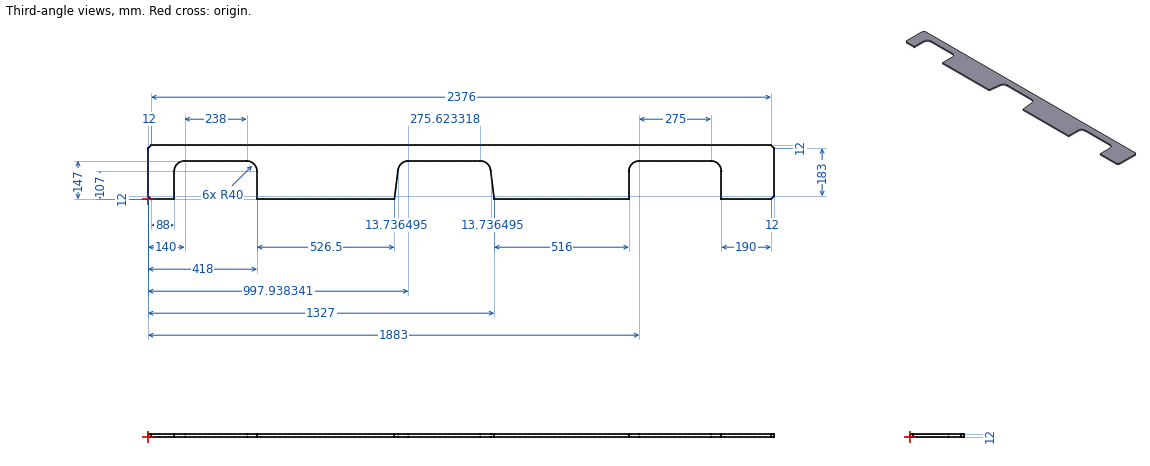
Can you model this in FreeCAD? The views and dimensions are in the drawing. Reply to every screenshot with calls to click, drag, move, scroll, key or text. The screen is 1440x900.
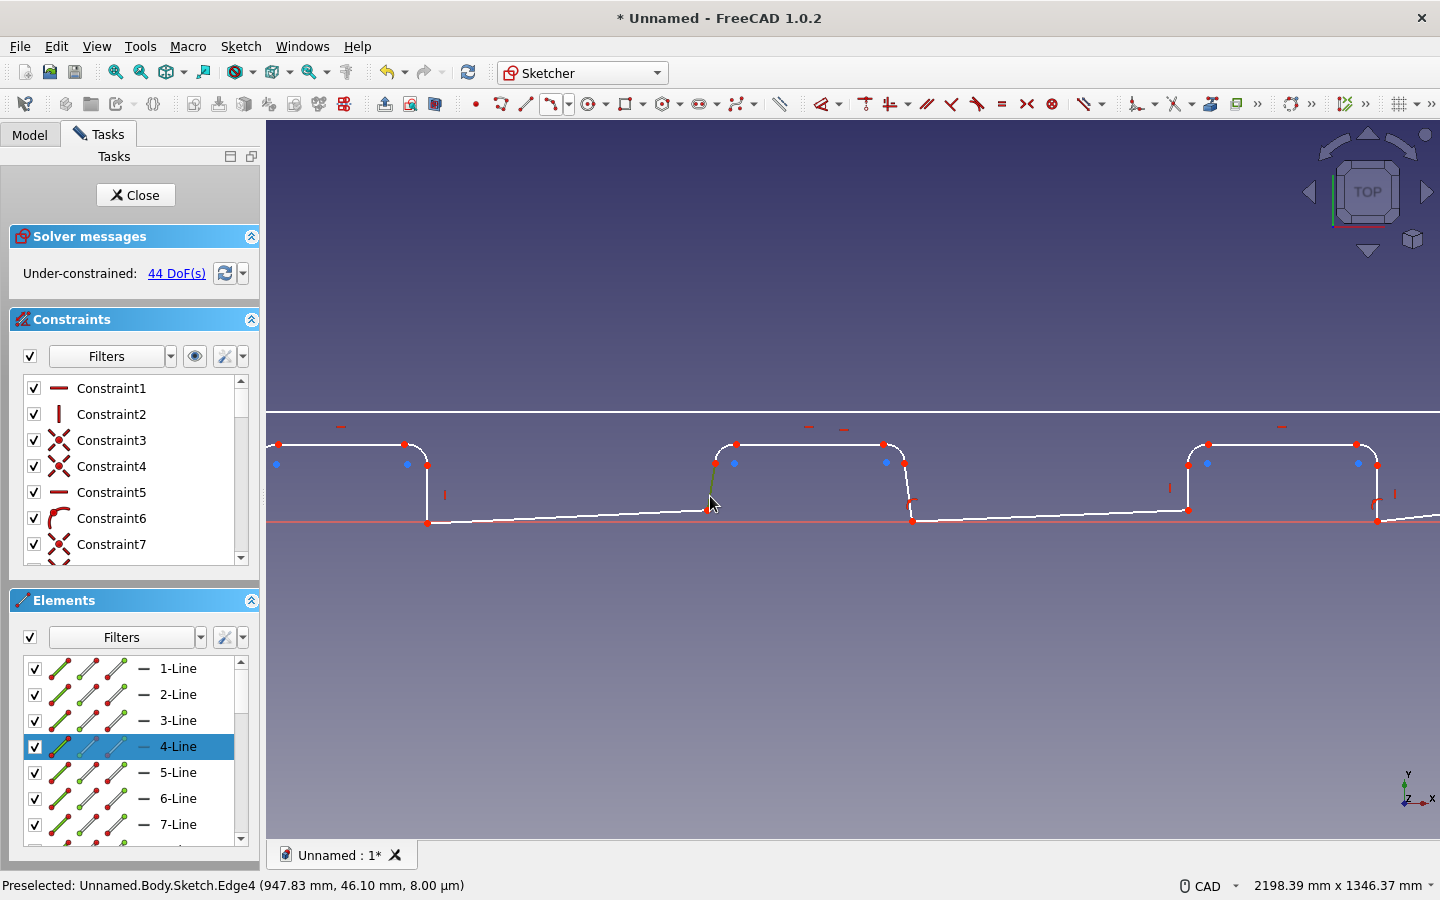
scroll(727, 446, up, 2)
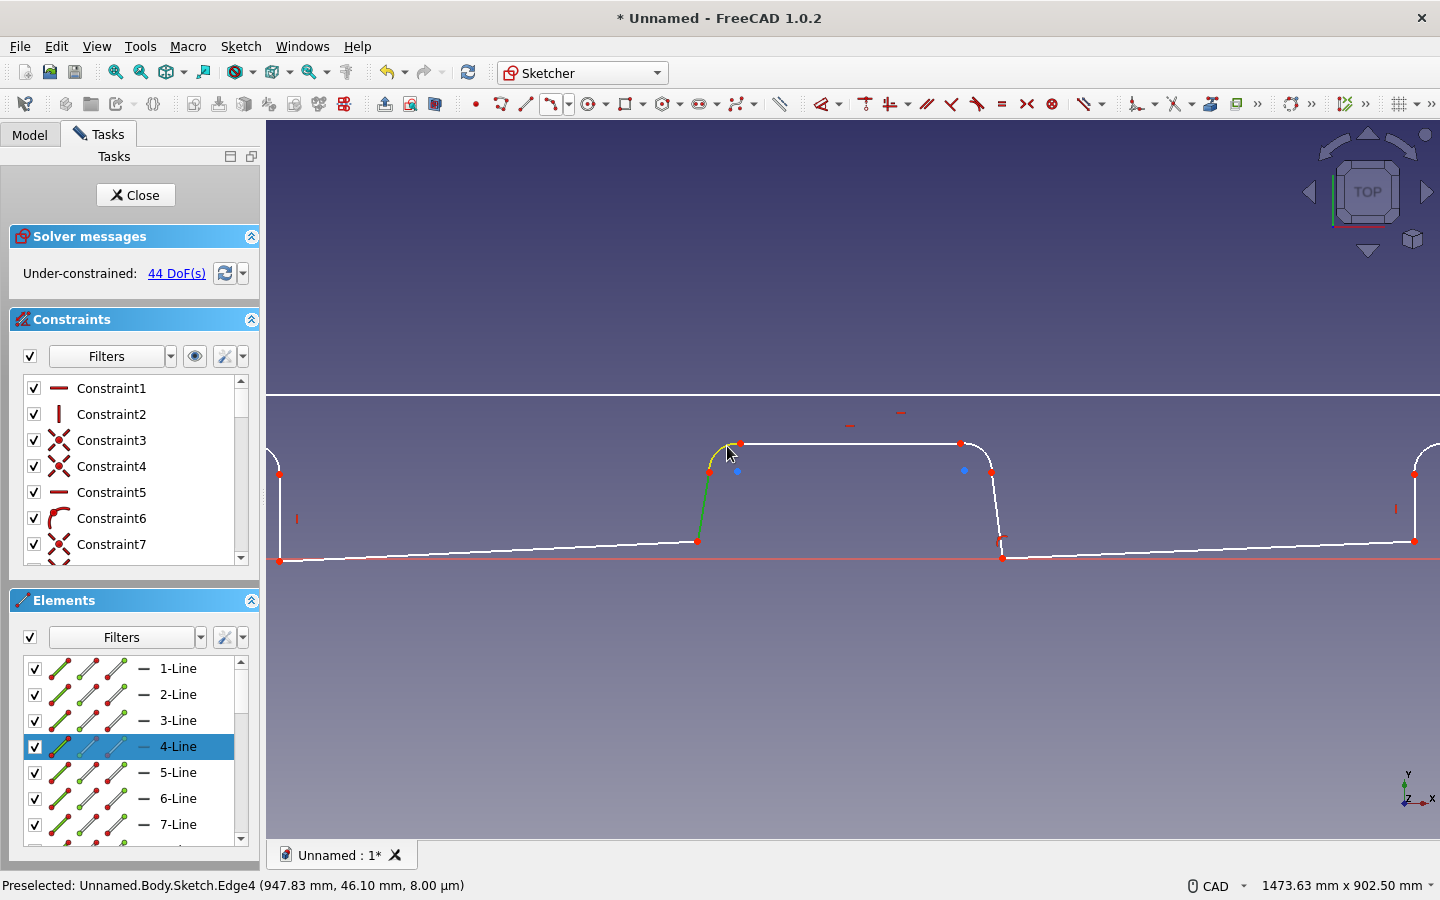
click(726, 446)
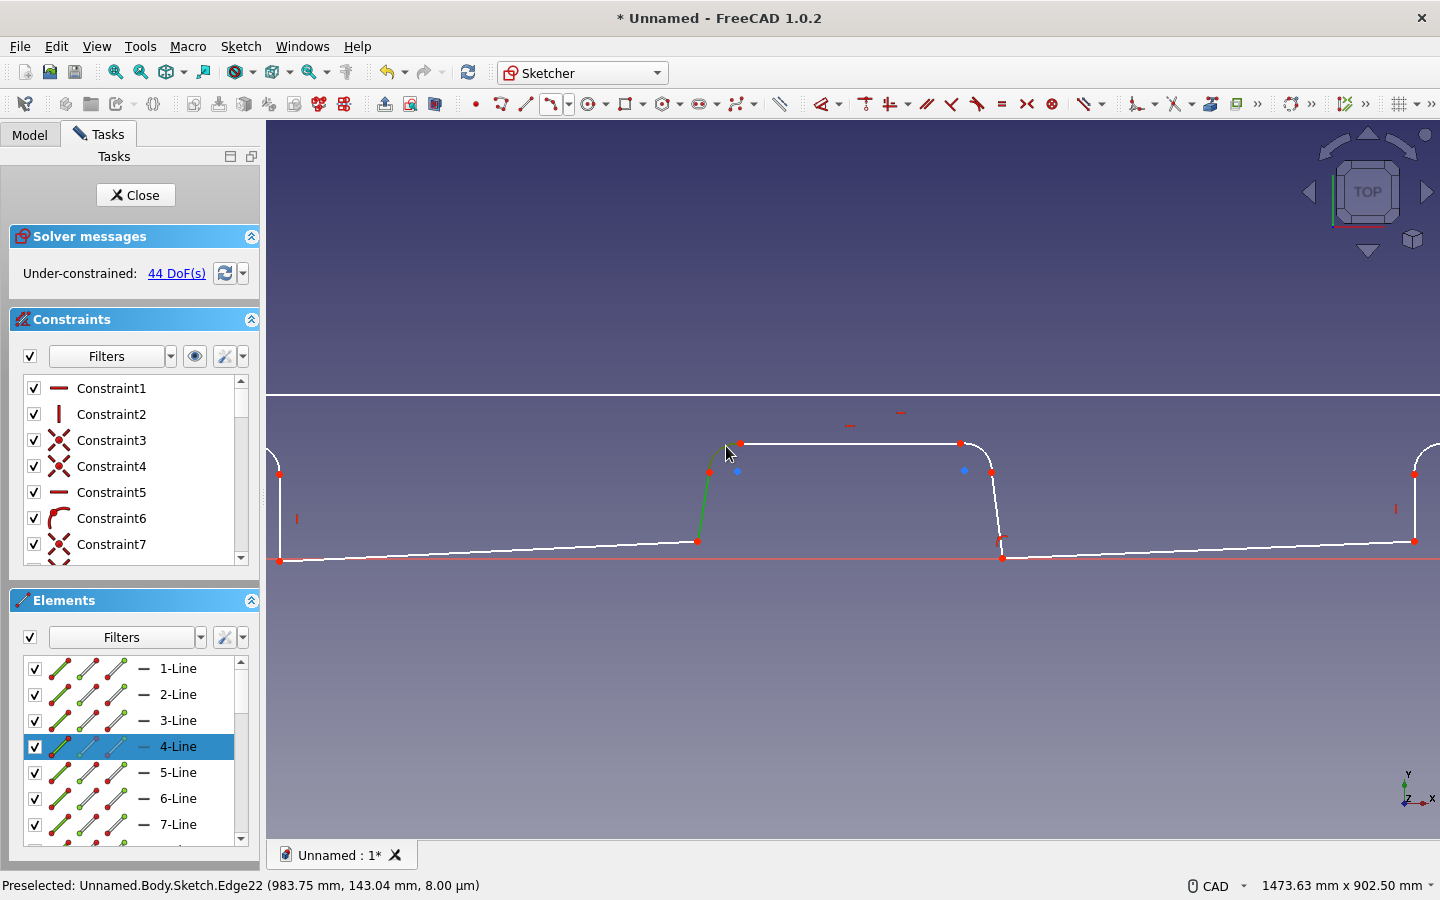
click(977, 104)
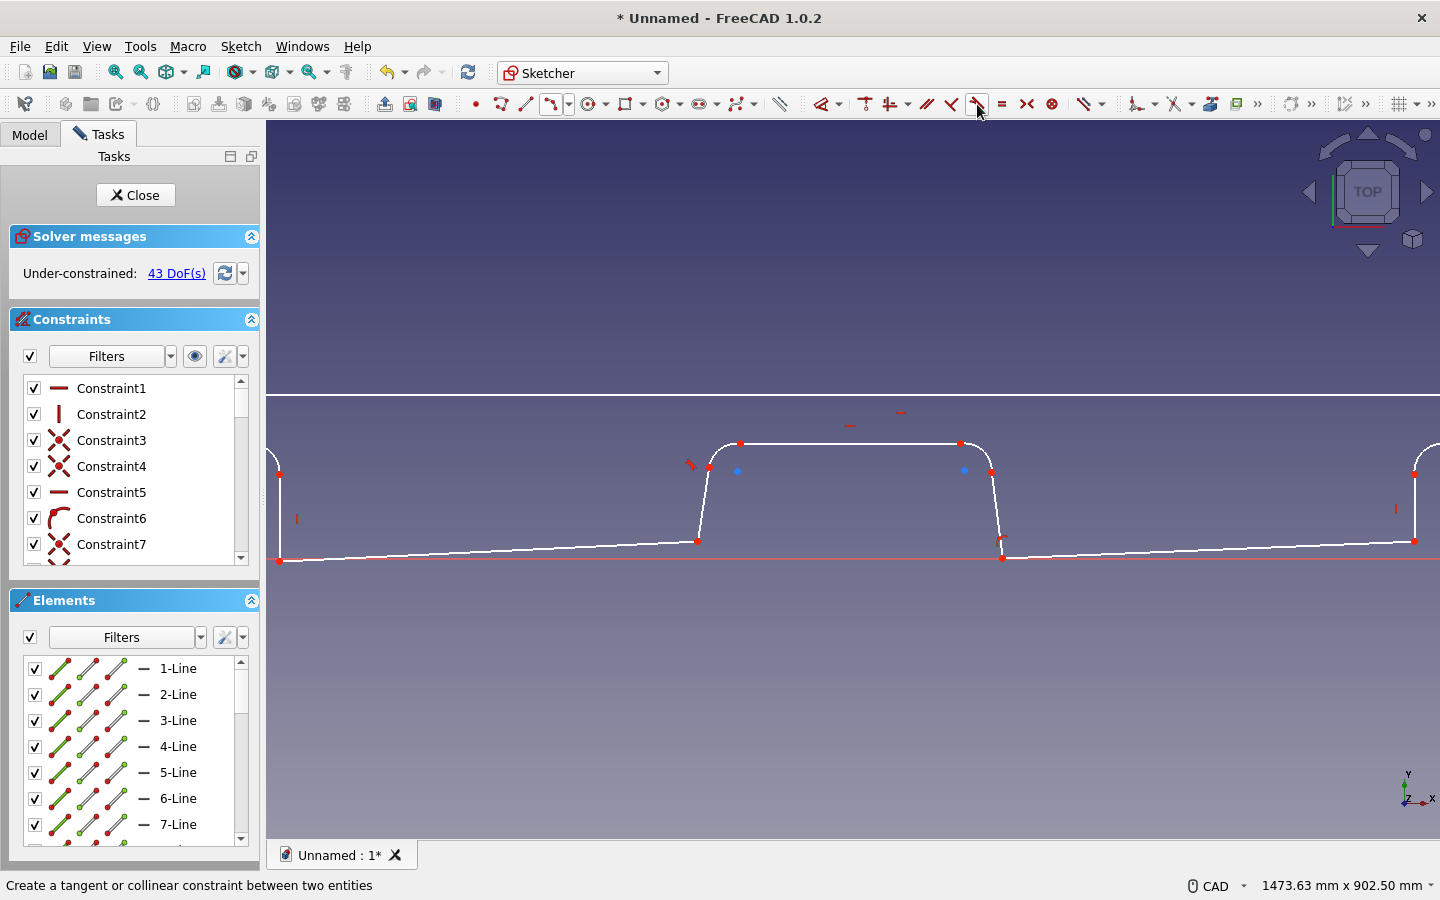
click(995, 498)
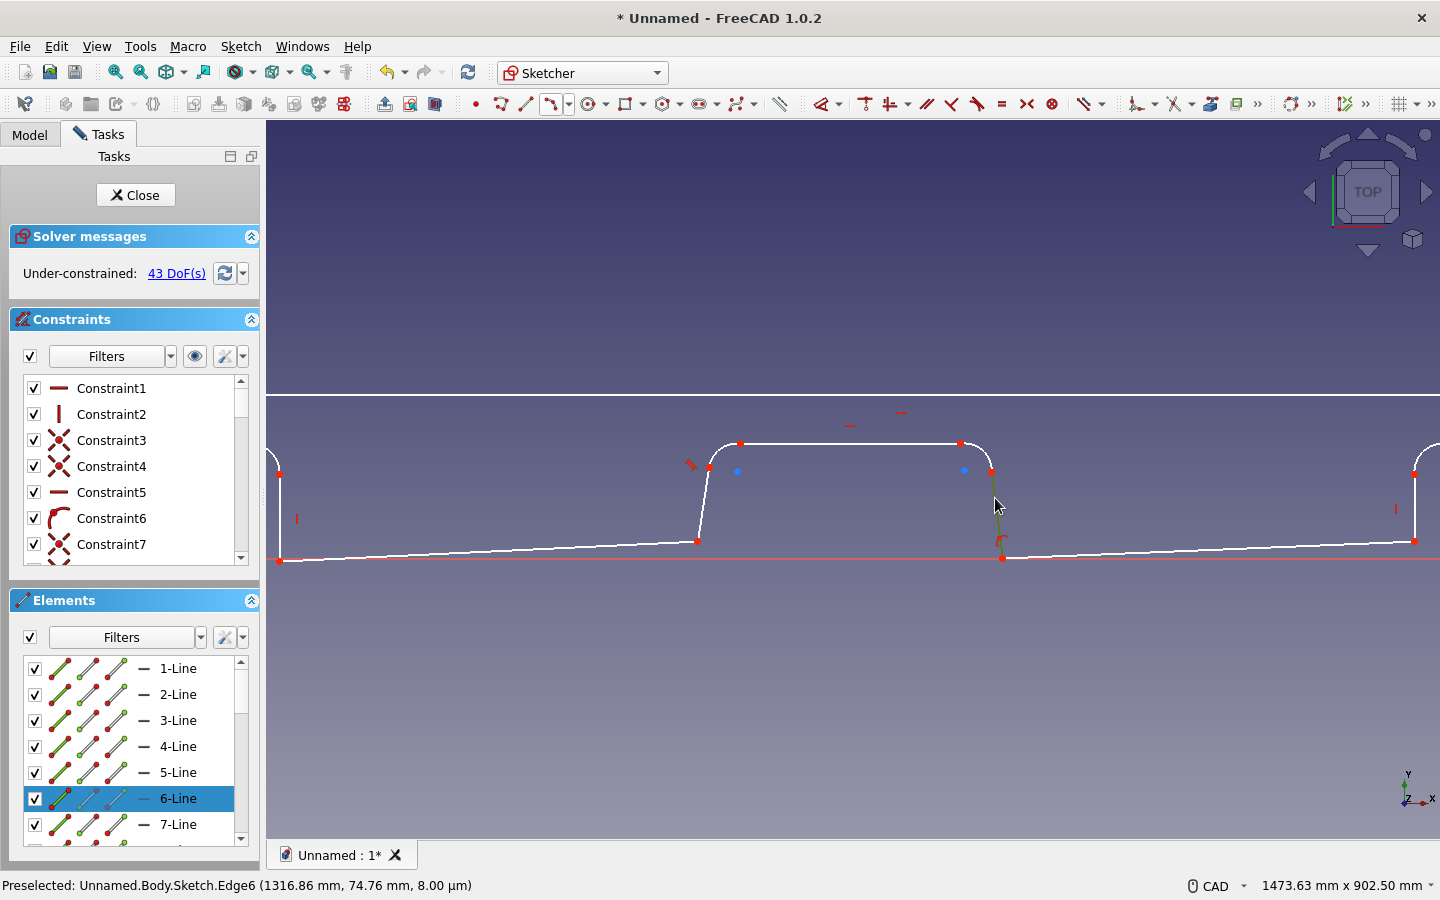
click(989, 458)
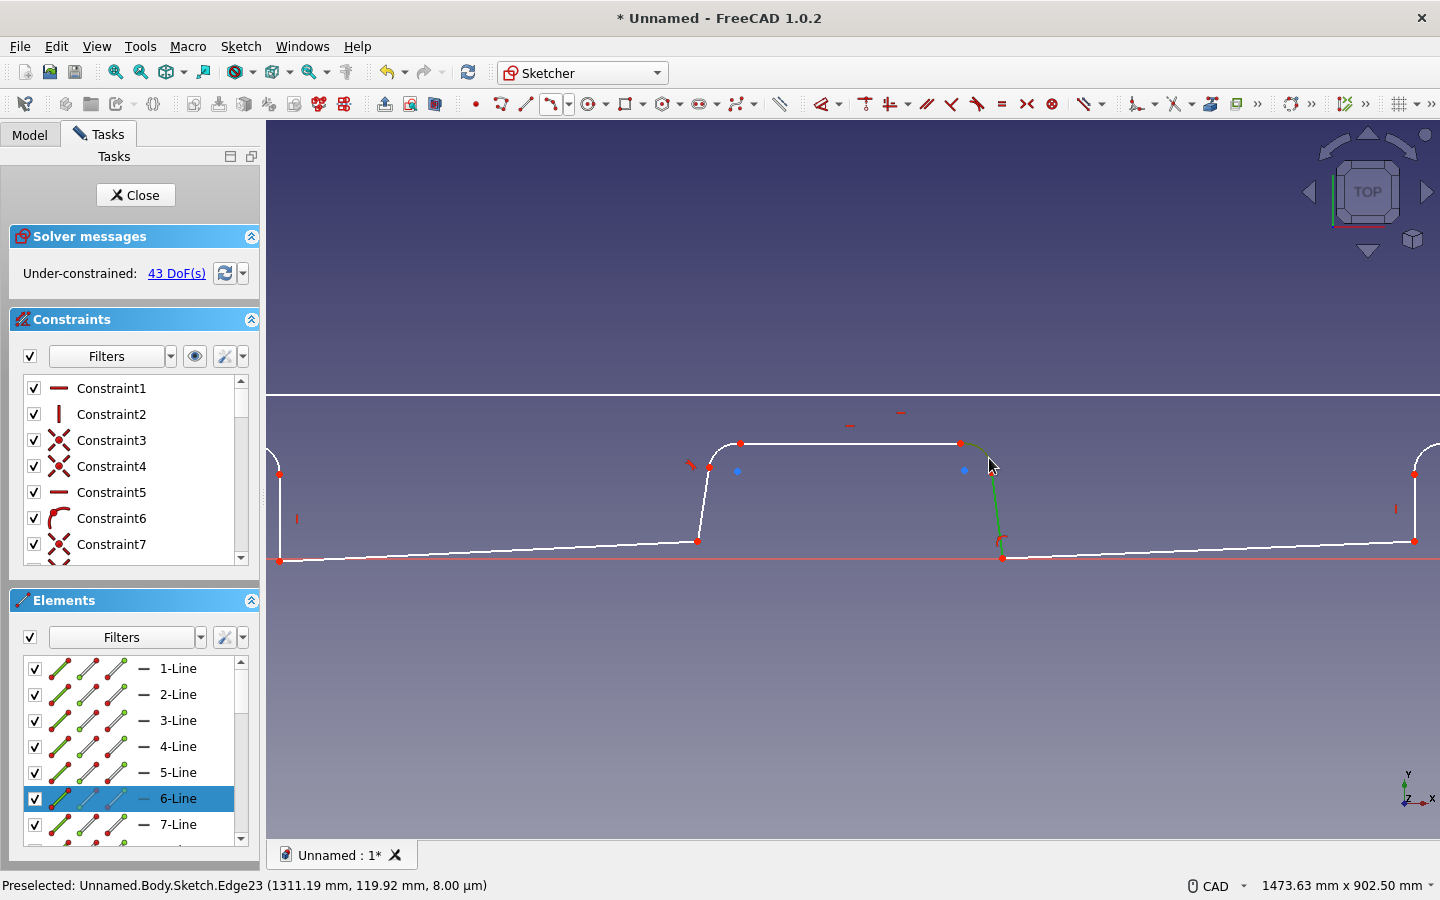
click(977, 104)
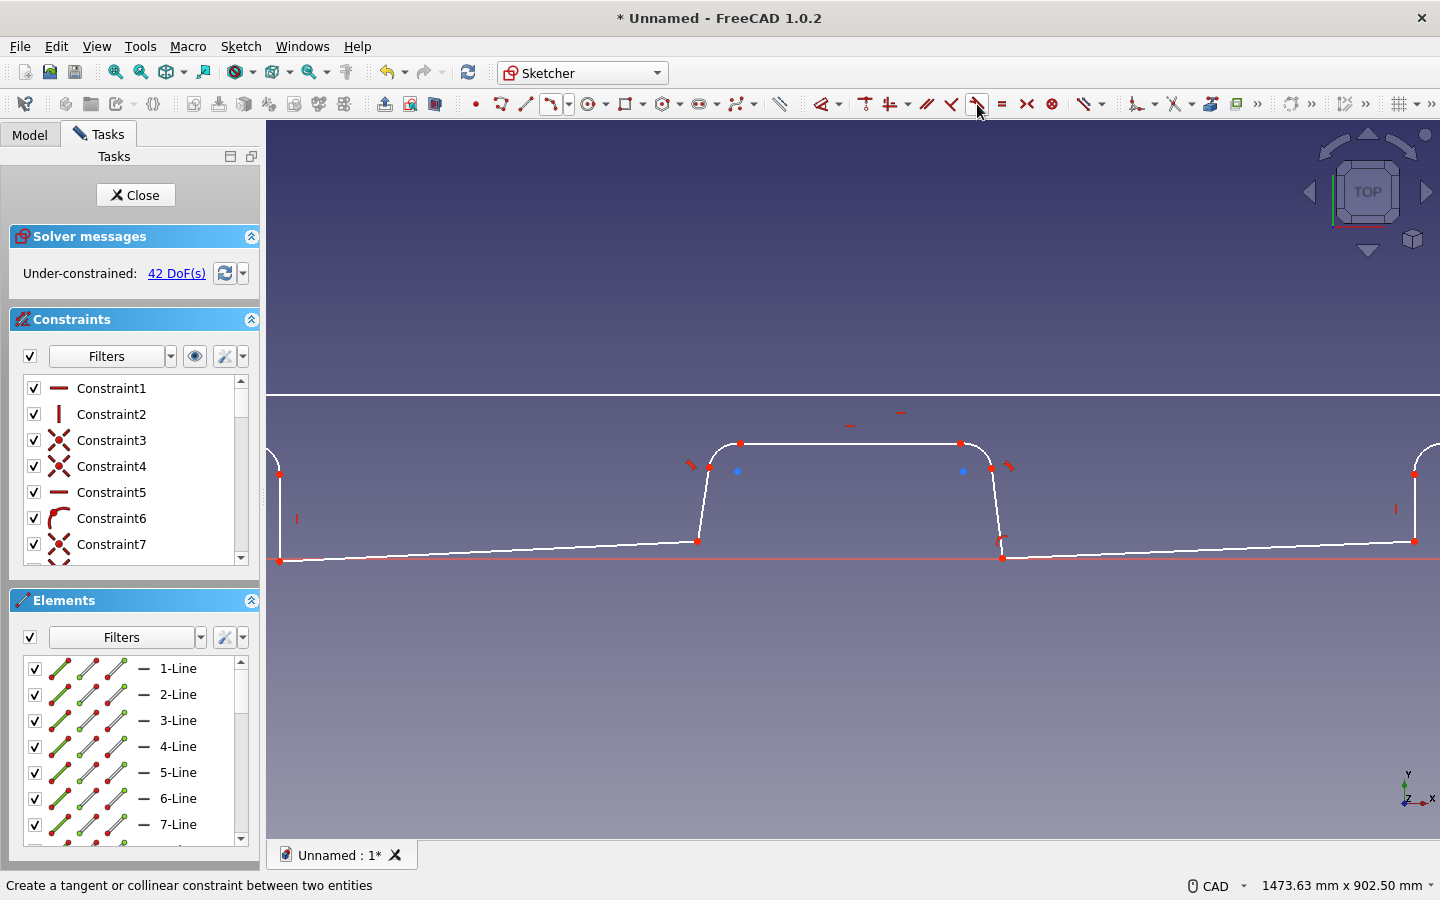
click(405, 556)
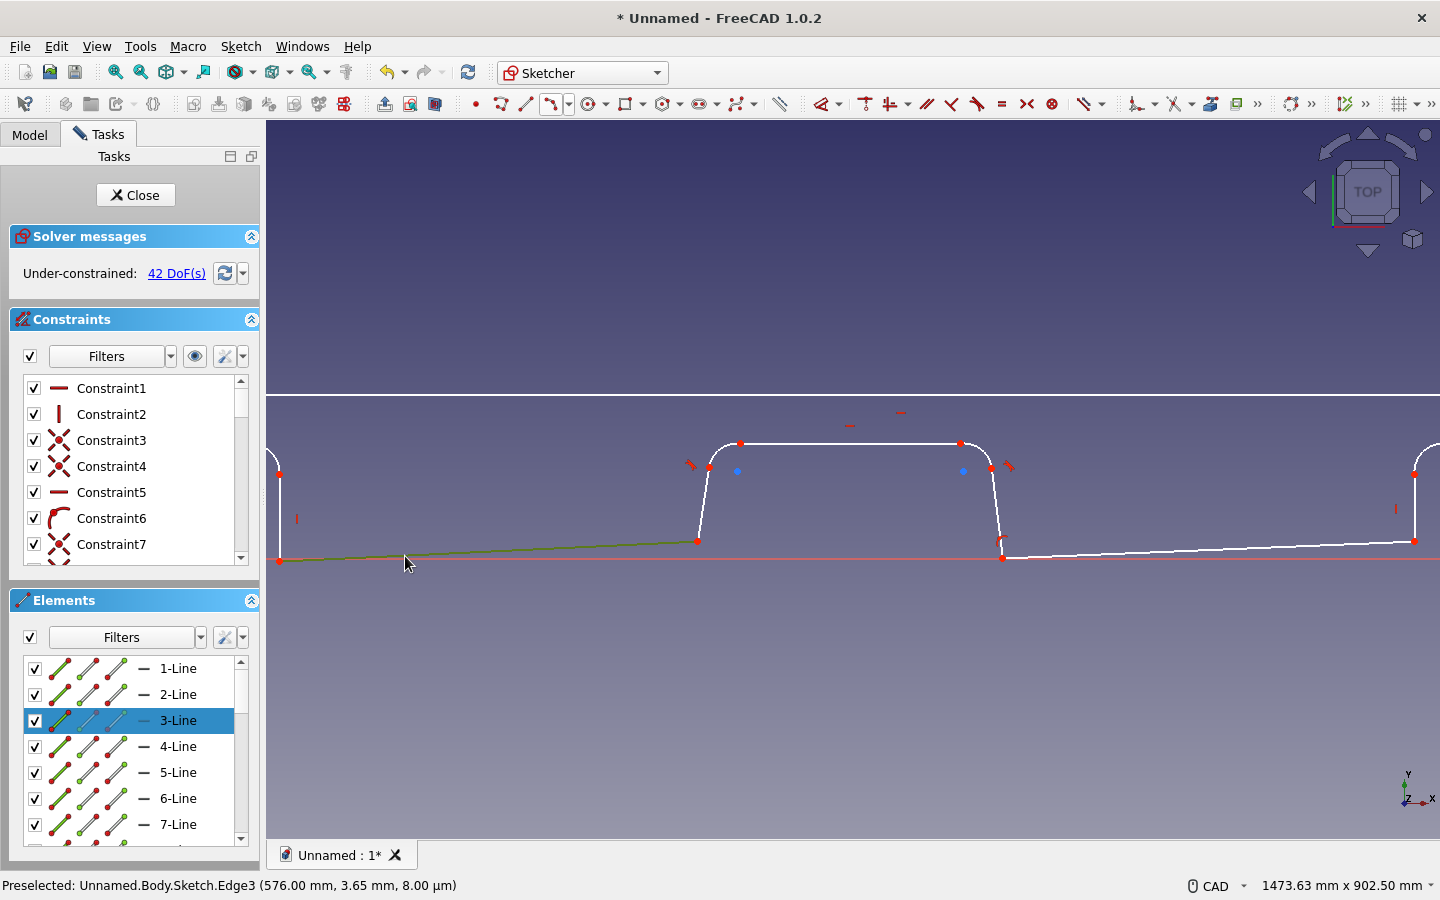
click(908, 104)